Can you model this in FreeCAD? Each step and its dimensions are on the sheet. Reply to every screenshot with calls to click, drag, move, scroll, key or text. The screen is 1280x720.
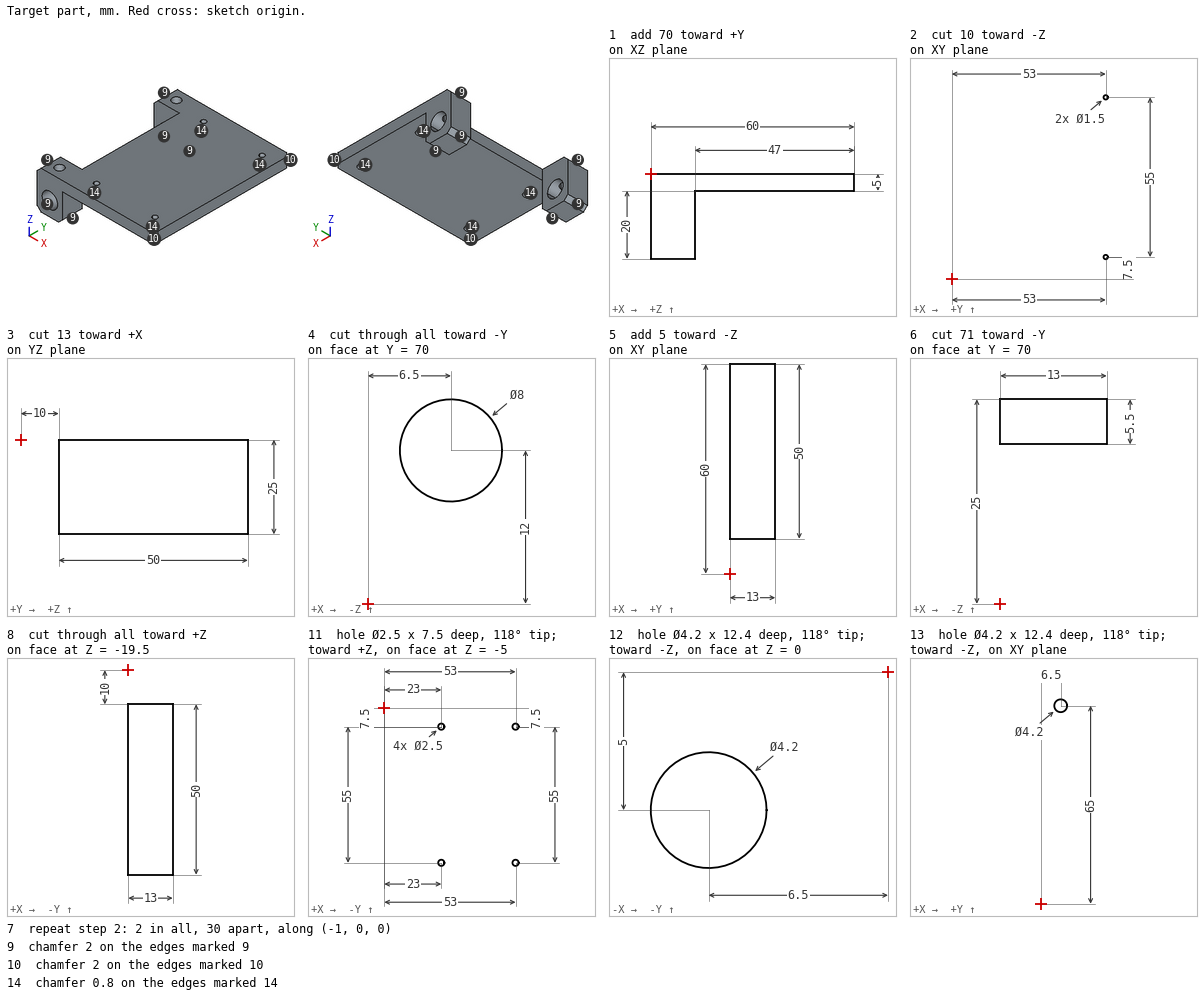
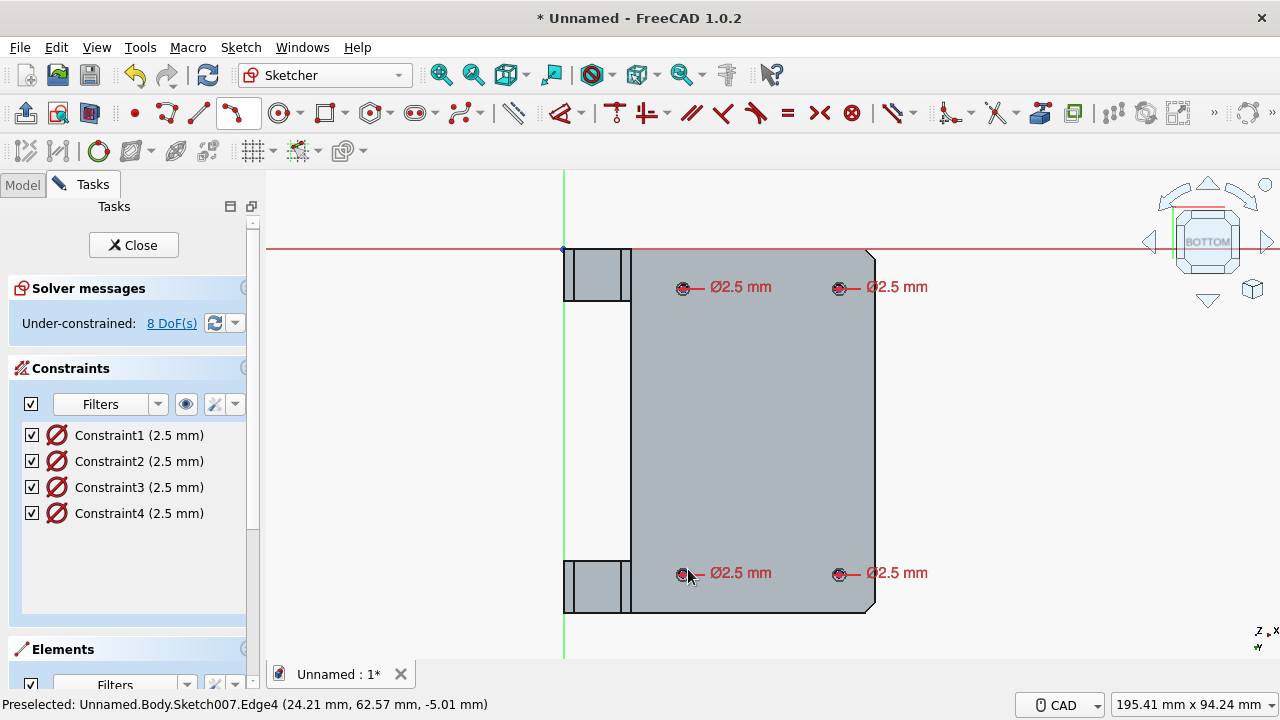
key(d)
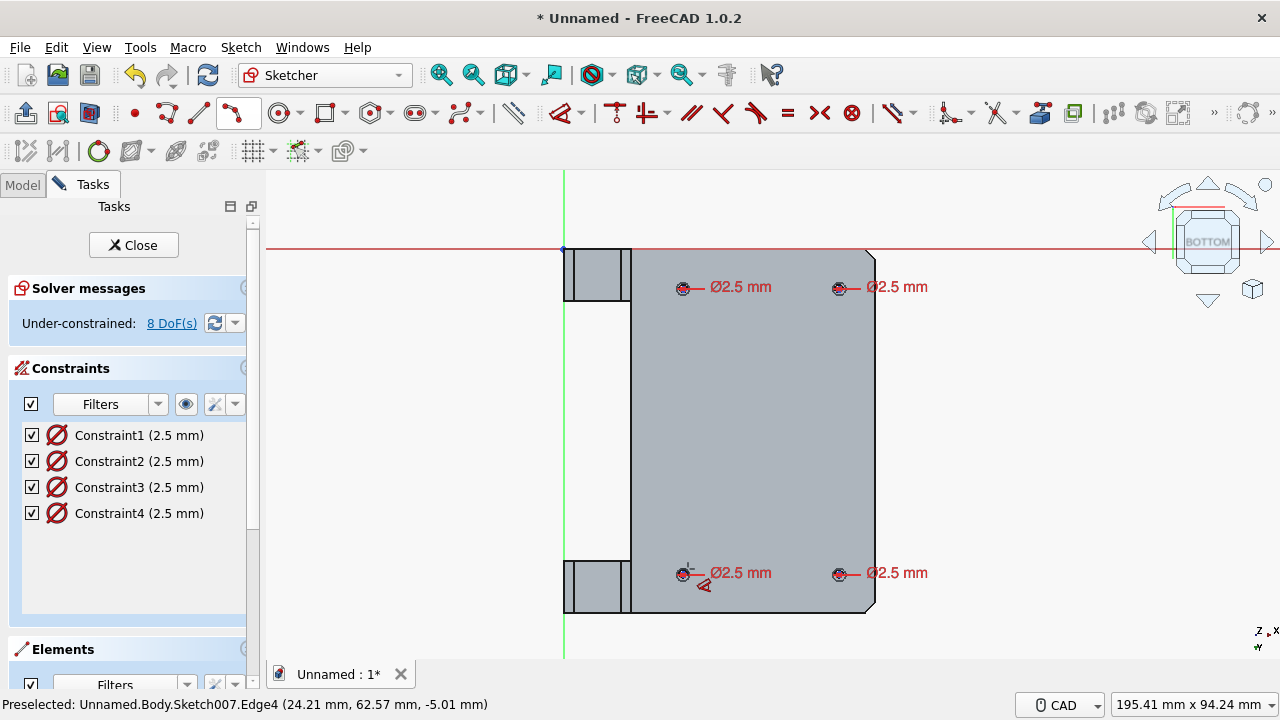
click(683, 289)
click(623, 215)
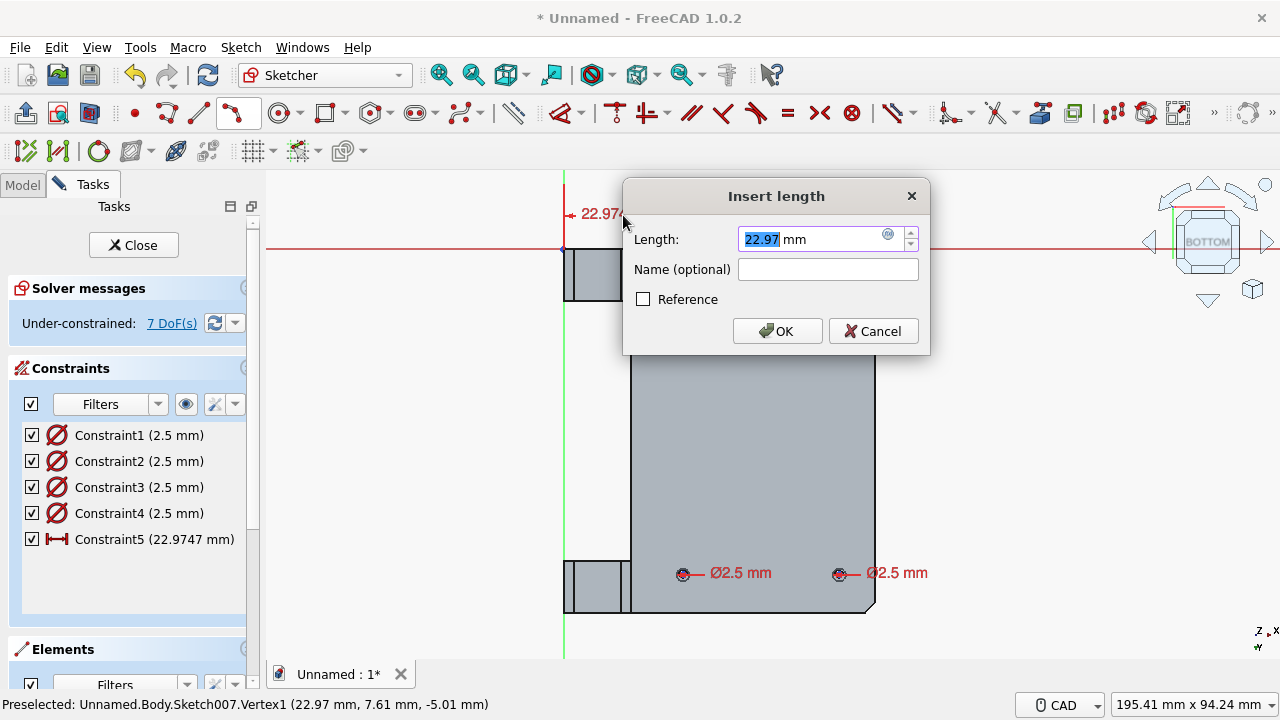
text(23)
key(Return)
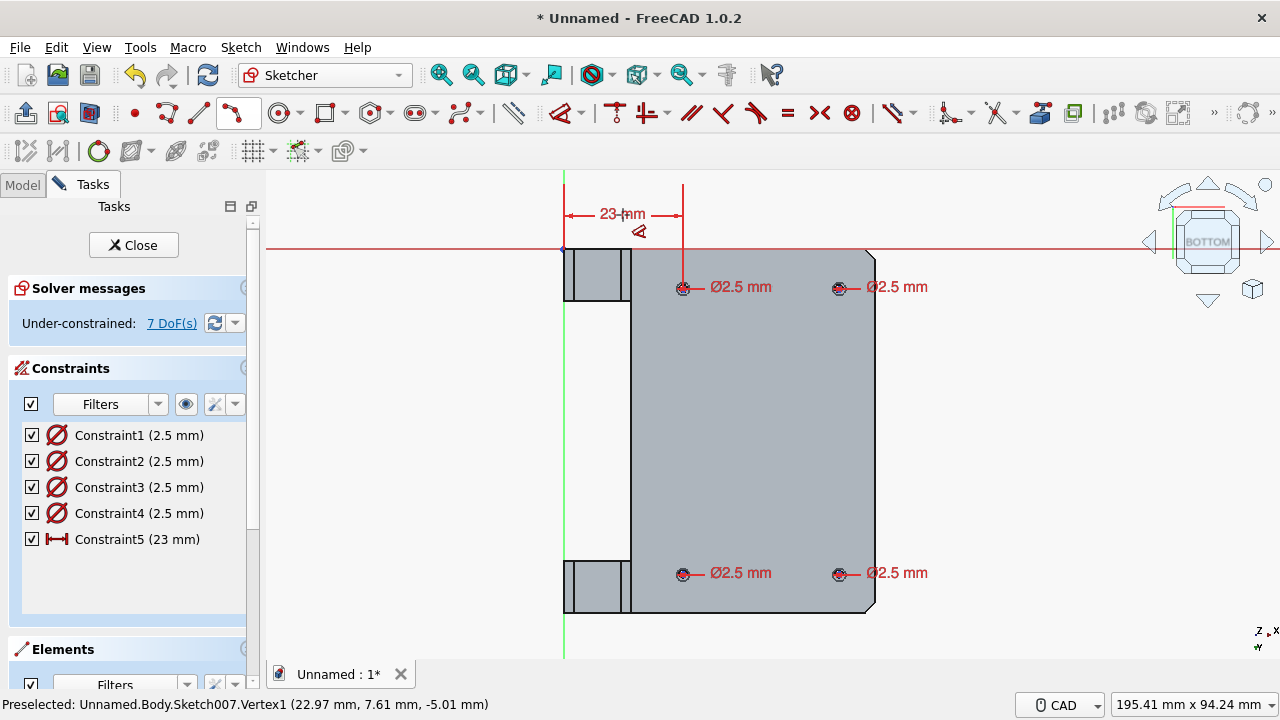
click(839, 289)
click(702, 215)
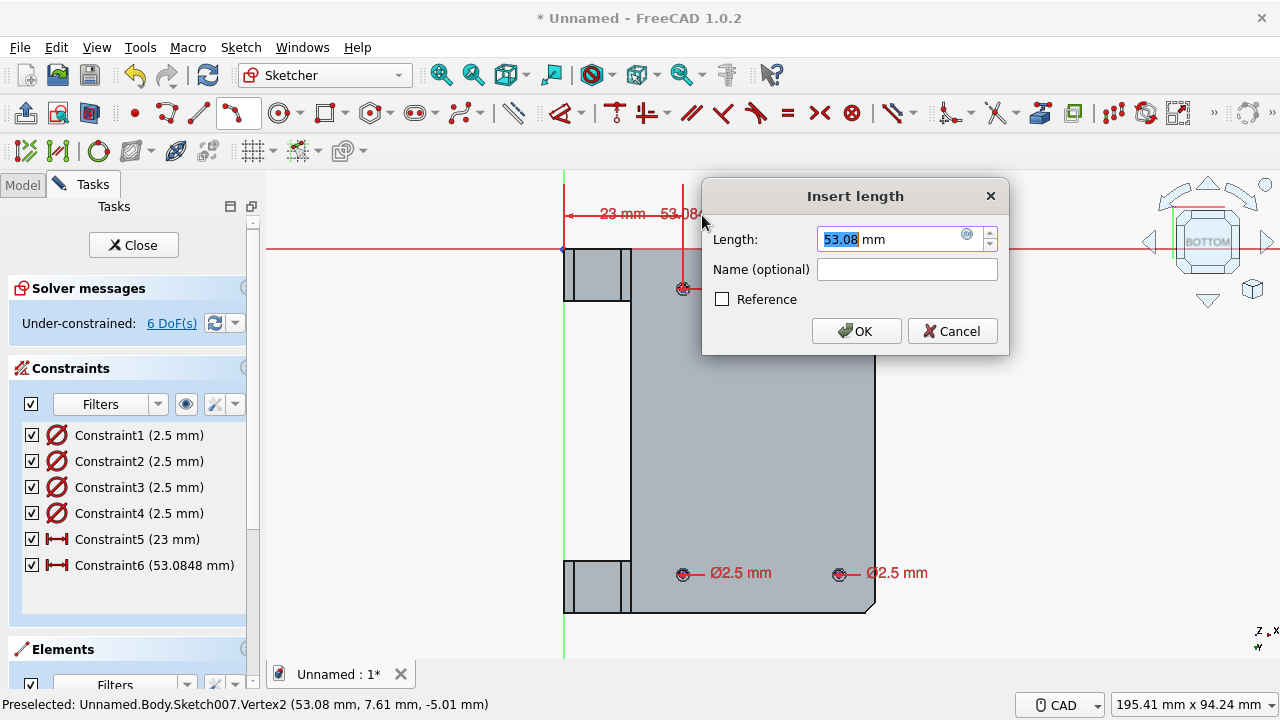
text(53)
key(Return)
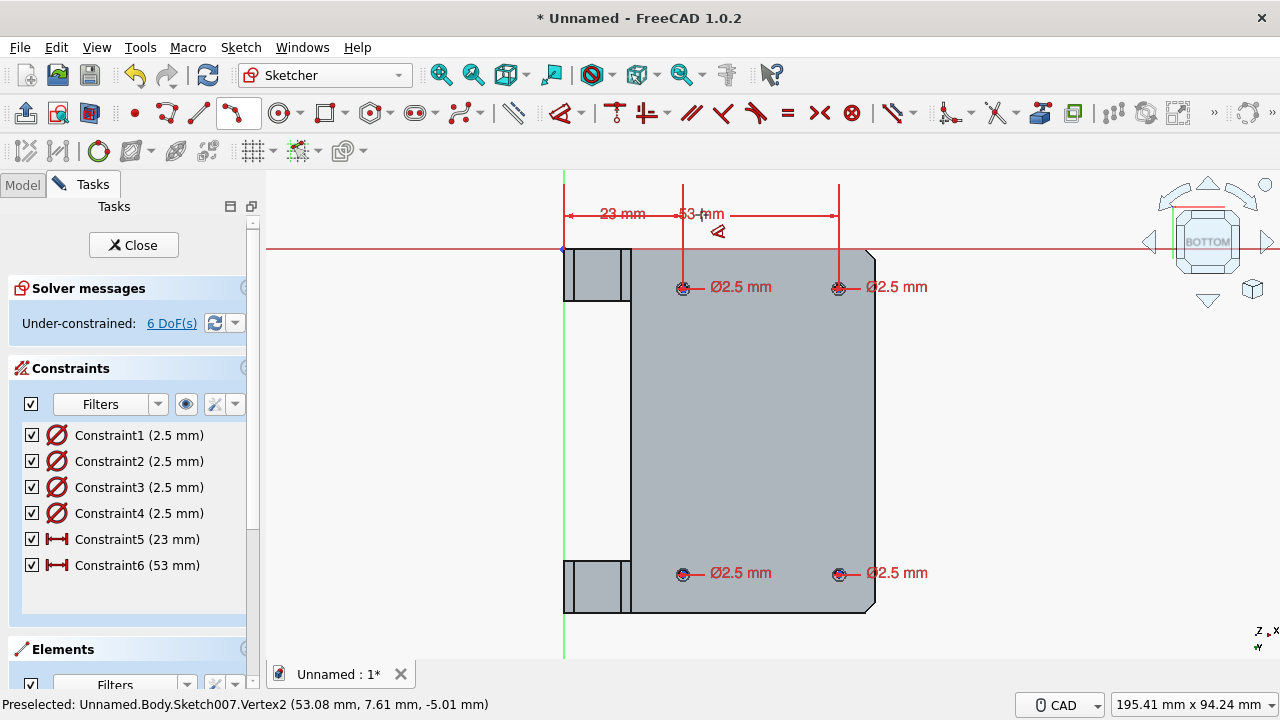
click(839, 575)
click(798, 215)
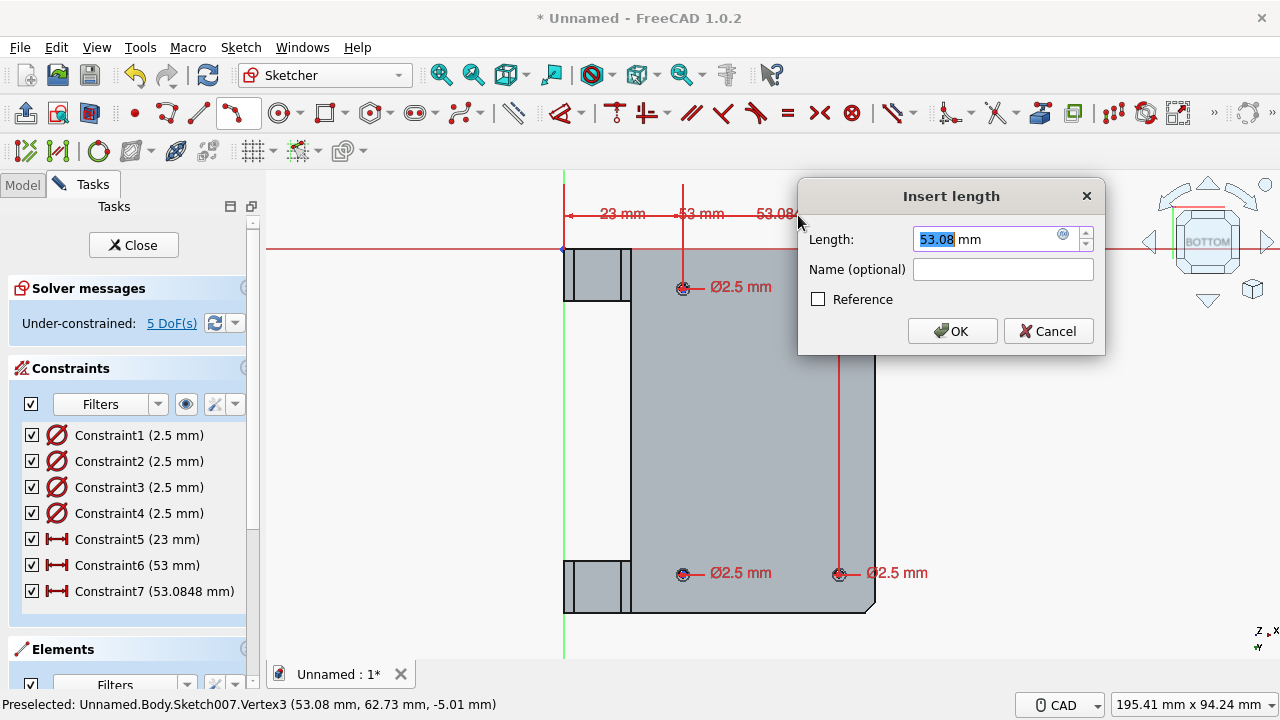
text(53)
key(Return)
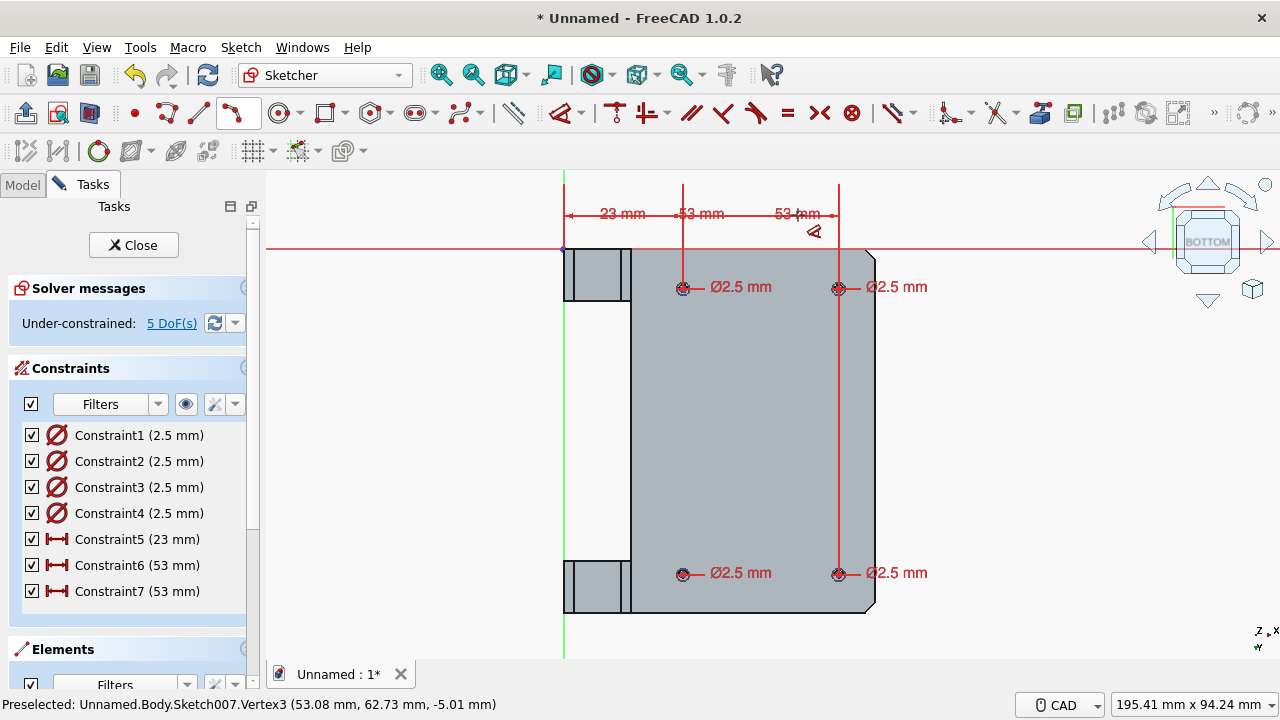
click(683, 575)
click(623, 609)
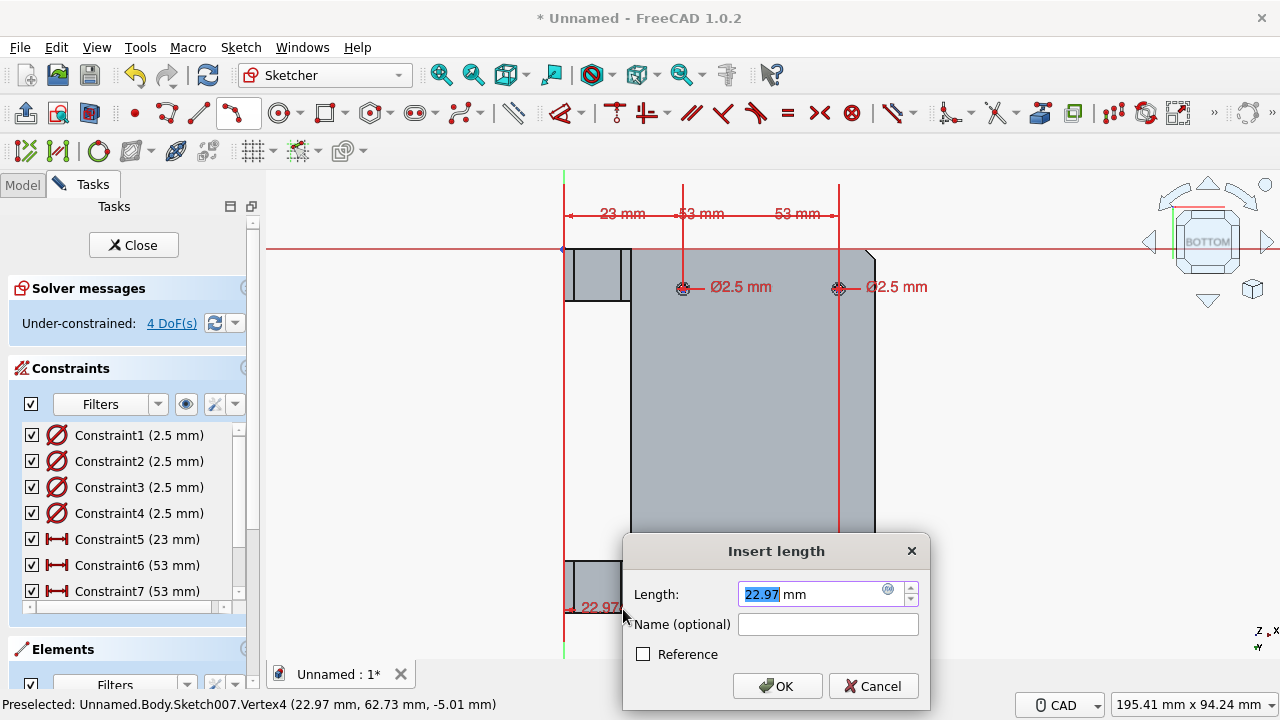
text(23)
key(Return)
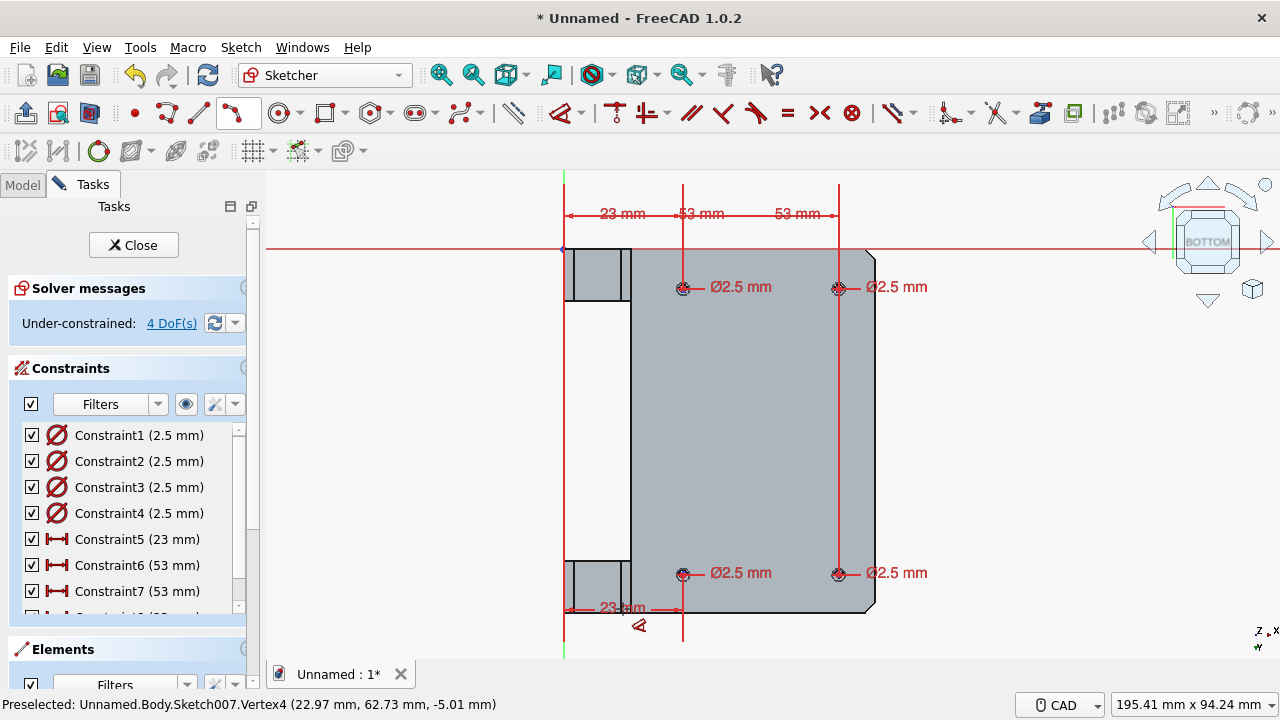
click(683, 289)
click(530, 269)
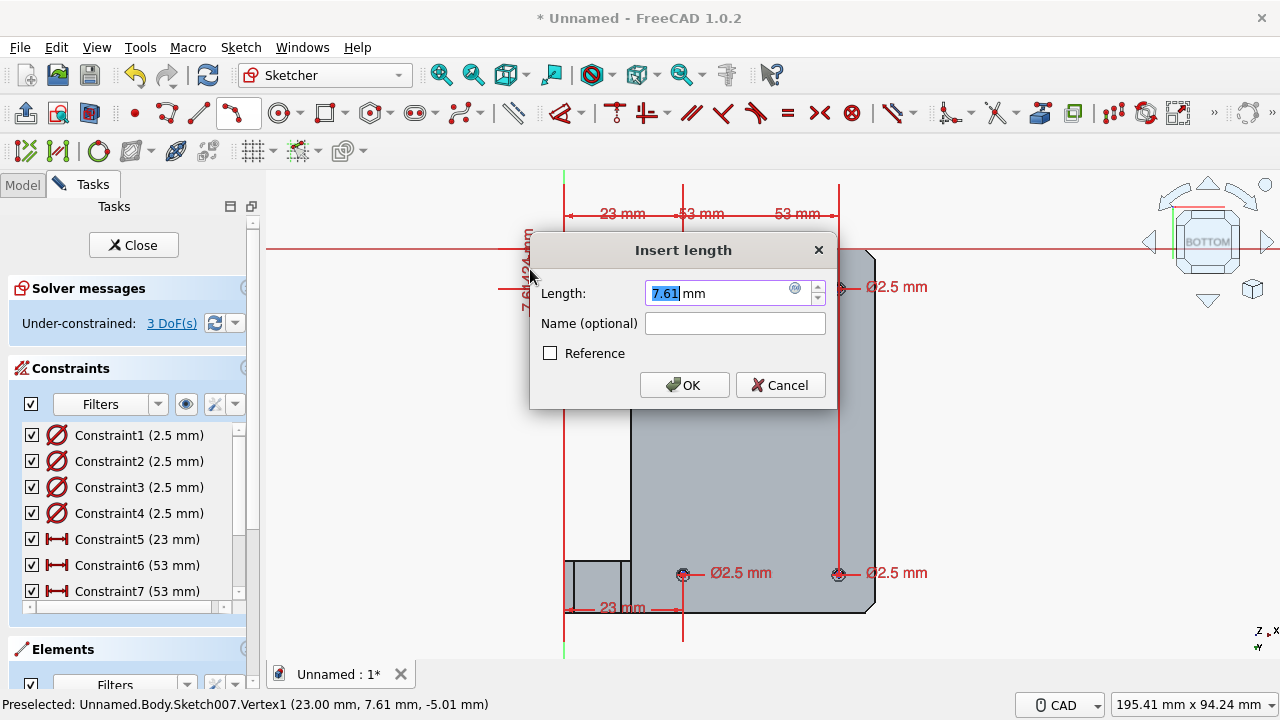
text(7.5)
key(Return)